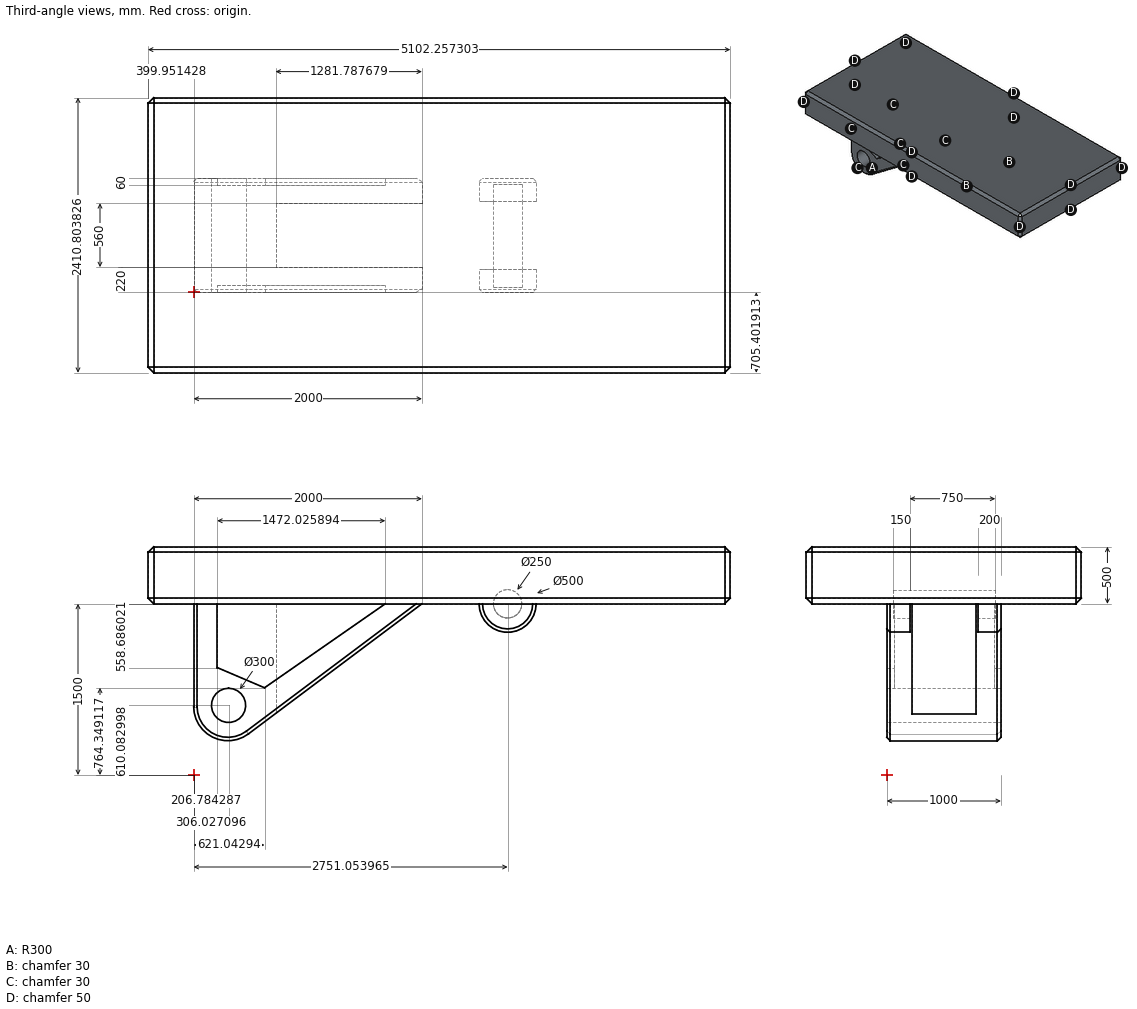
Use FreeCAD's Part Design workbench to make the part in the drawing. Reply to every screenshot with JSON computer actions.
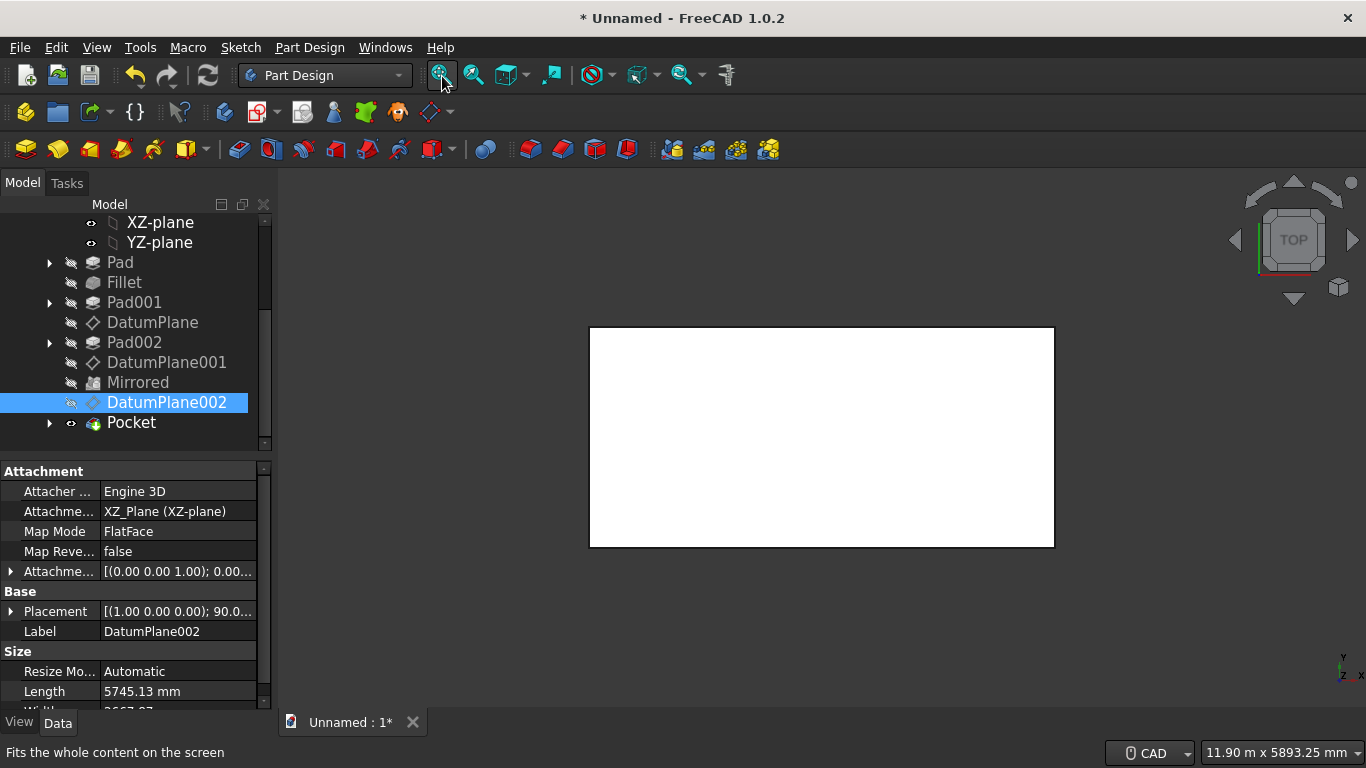
{"action": "key", "text": "0"}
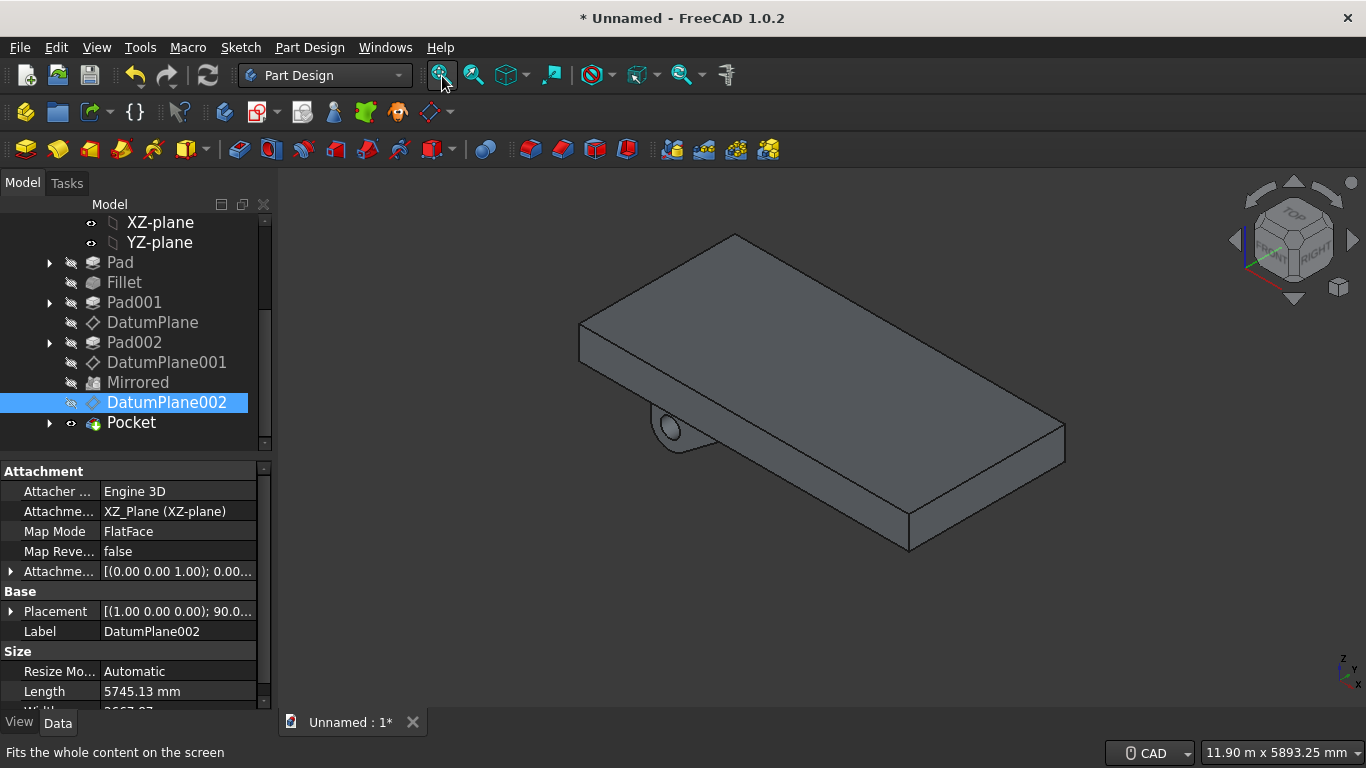
{"action": "key", "text": "1"}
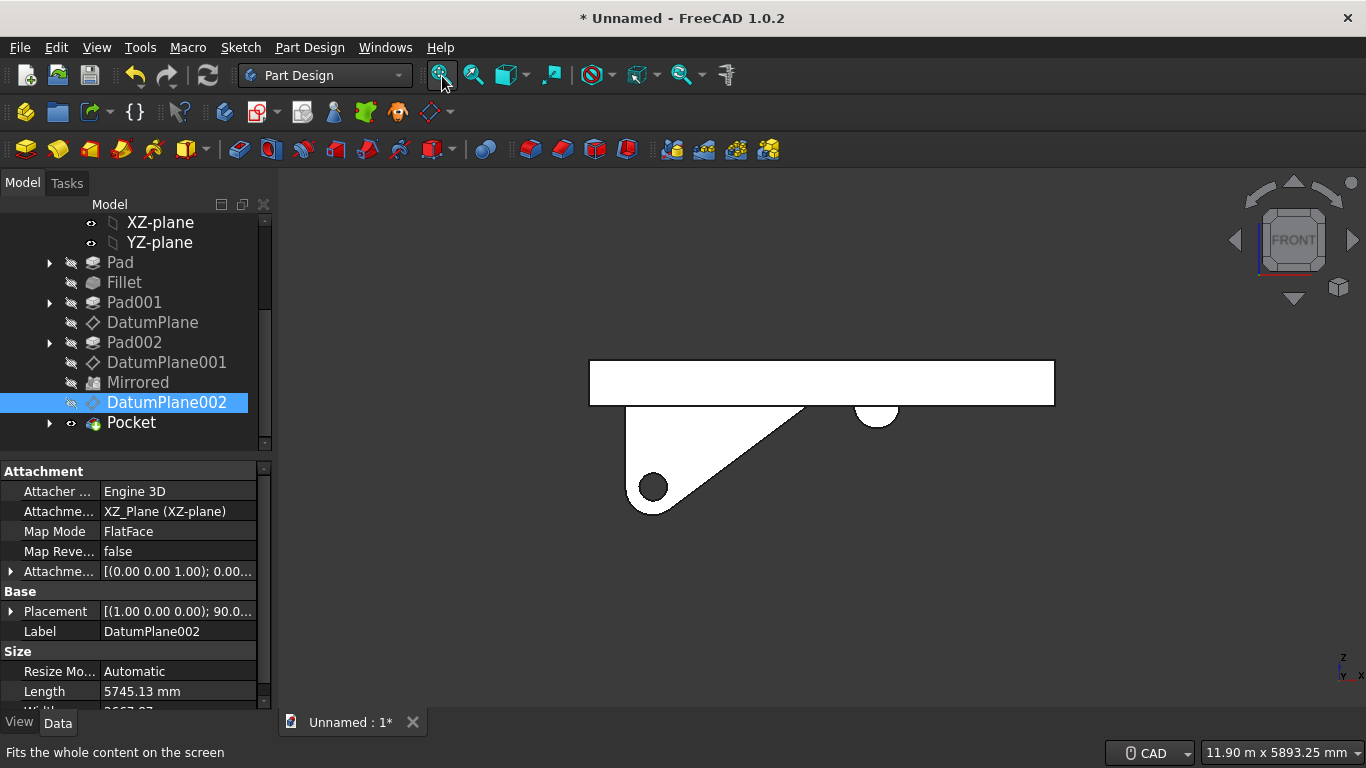
{"action": "left_click", "coordinate": [442, 76]}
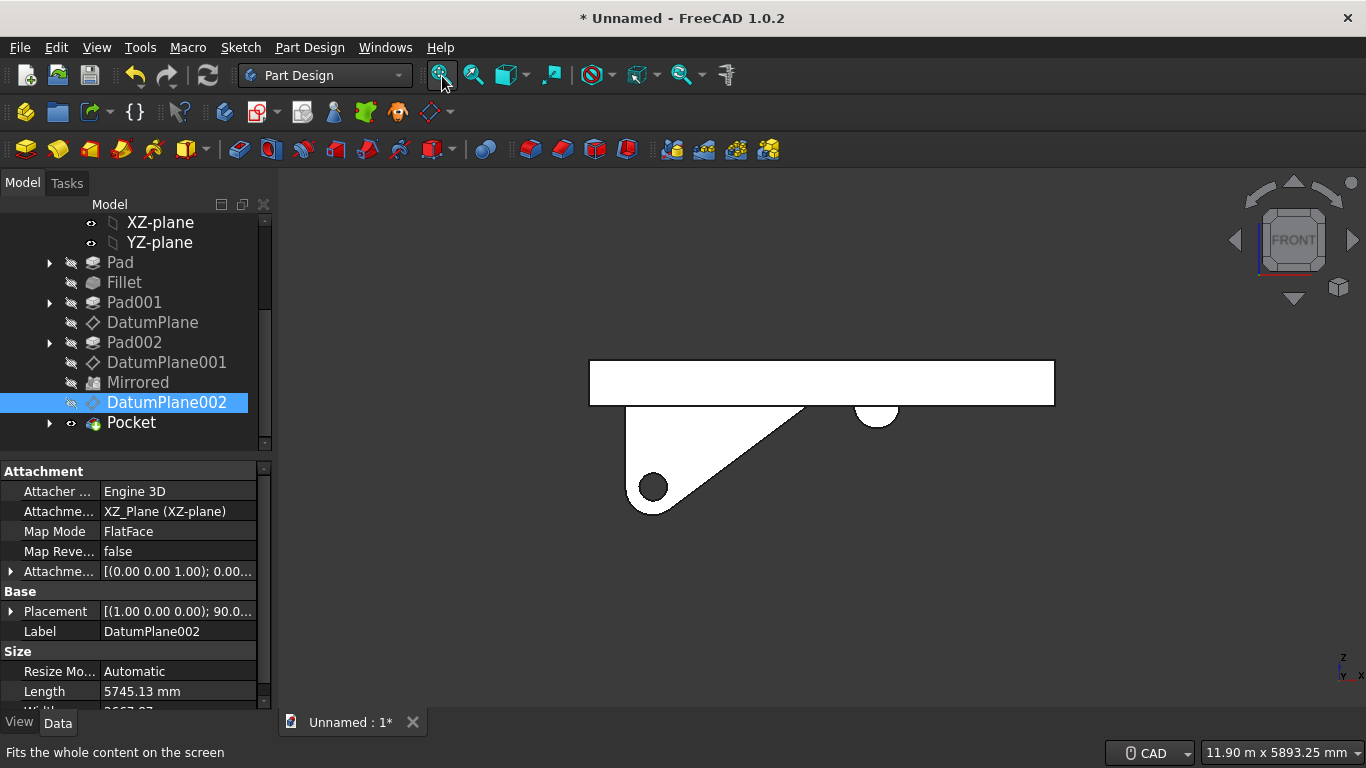
{"action": "left_click", "coordinate": [863, 423]}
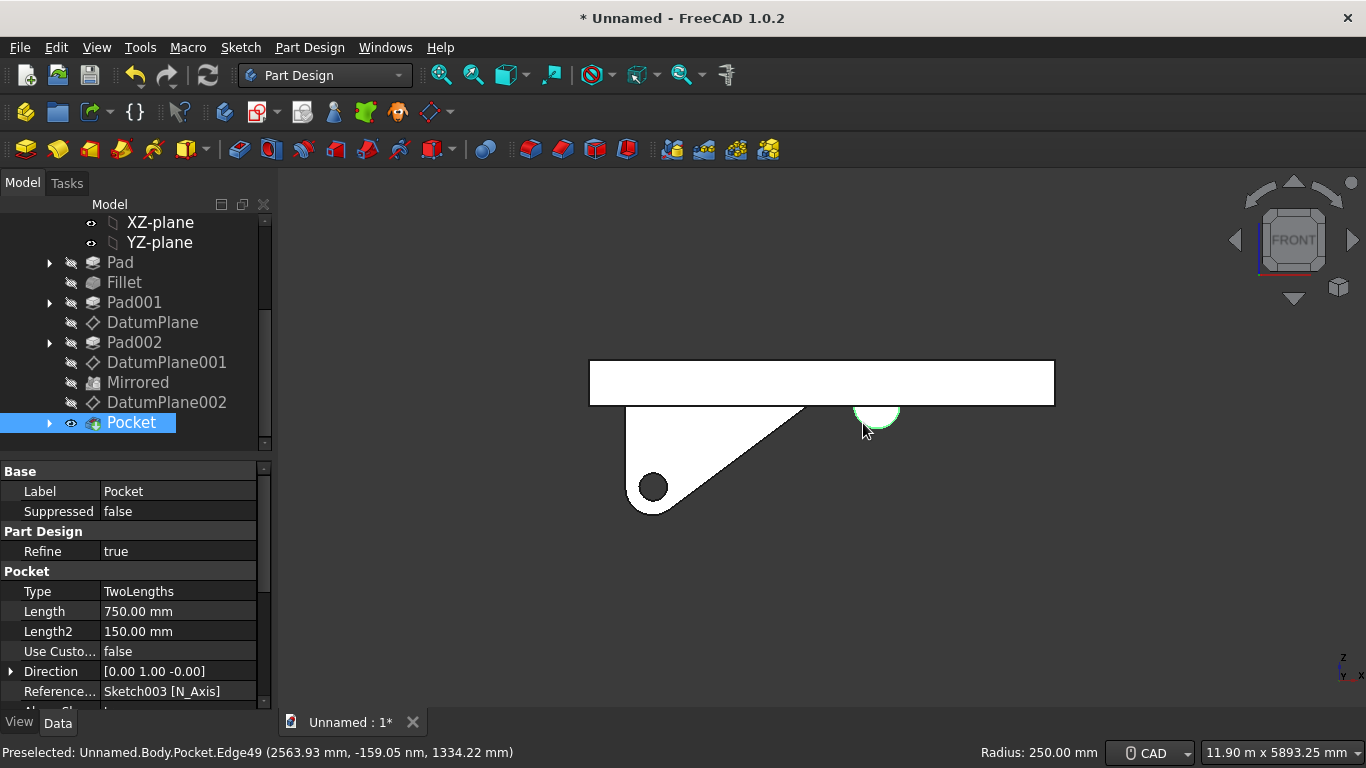
{"action": "key", "text": "3"}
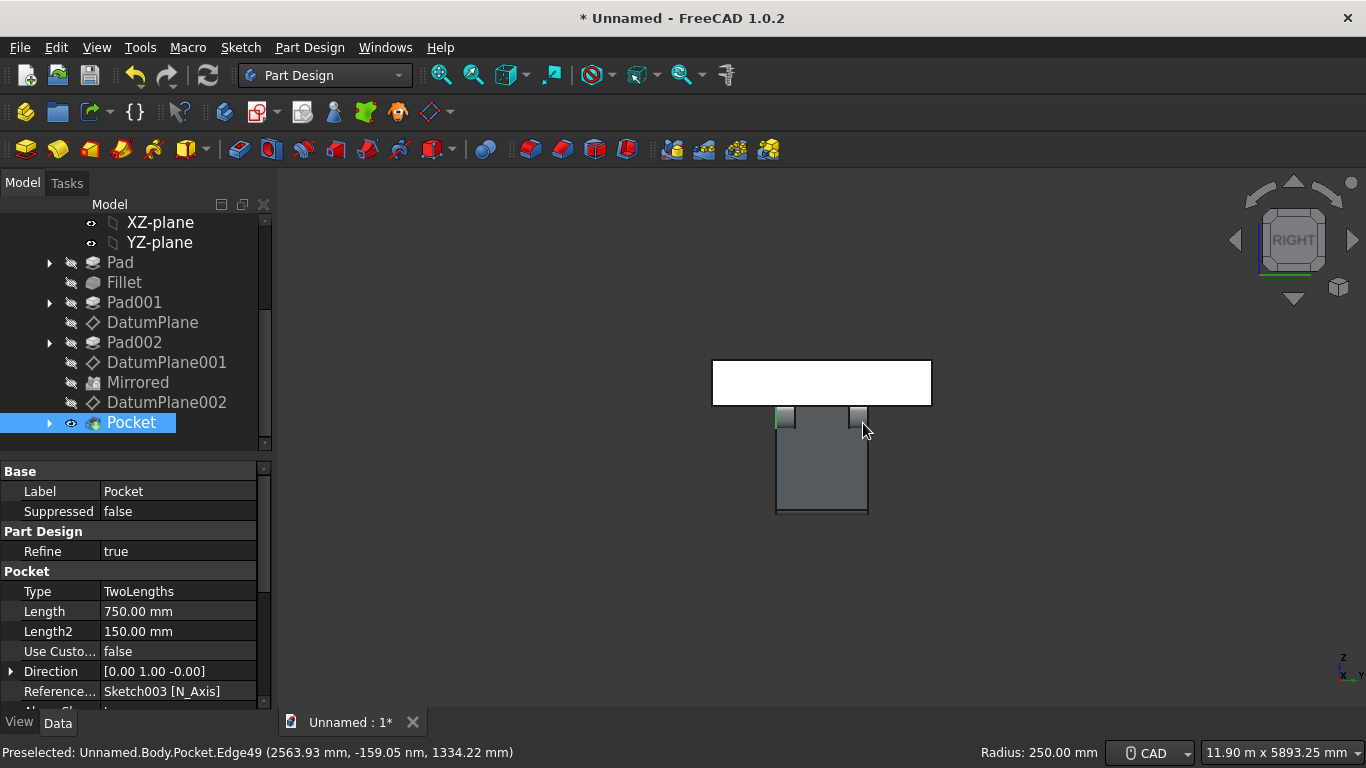
{"action": "key", "text": "v f"}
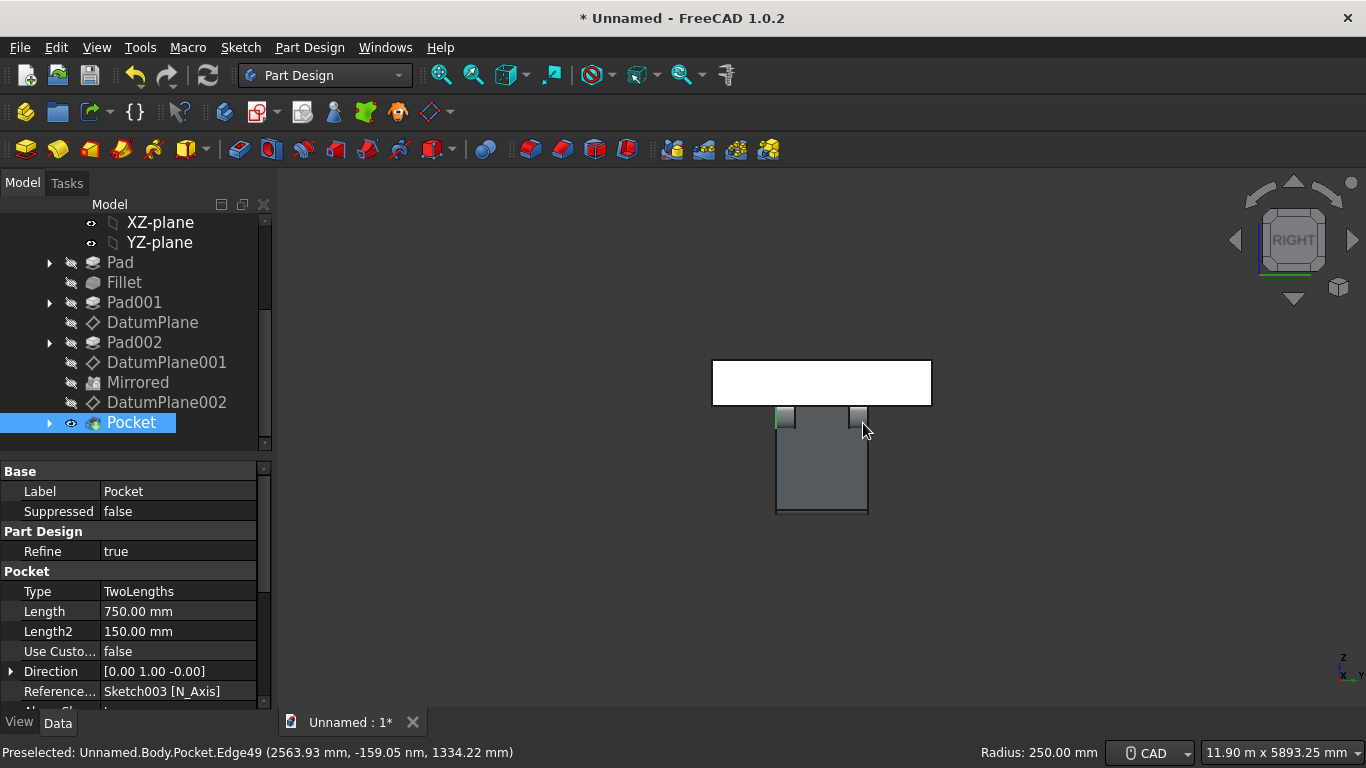
{"action": "left_click", "coordinate": [868, 427], "text": "ctrl"}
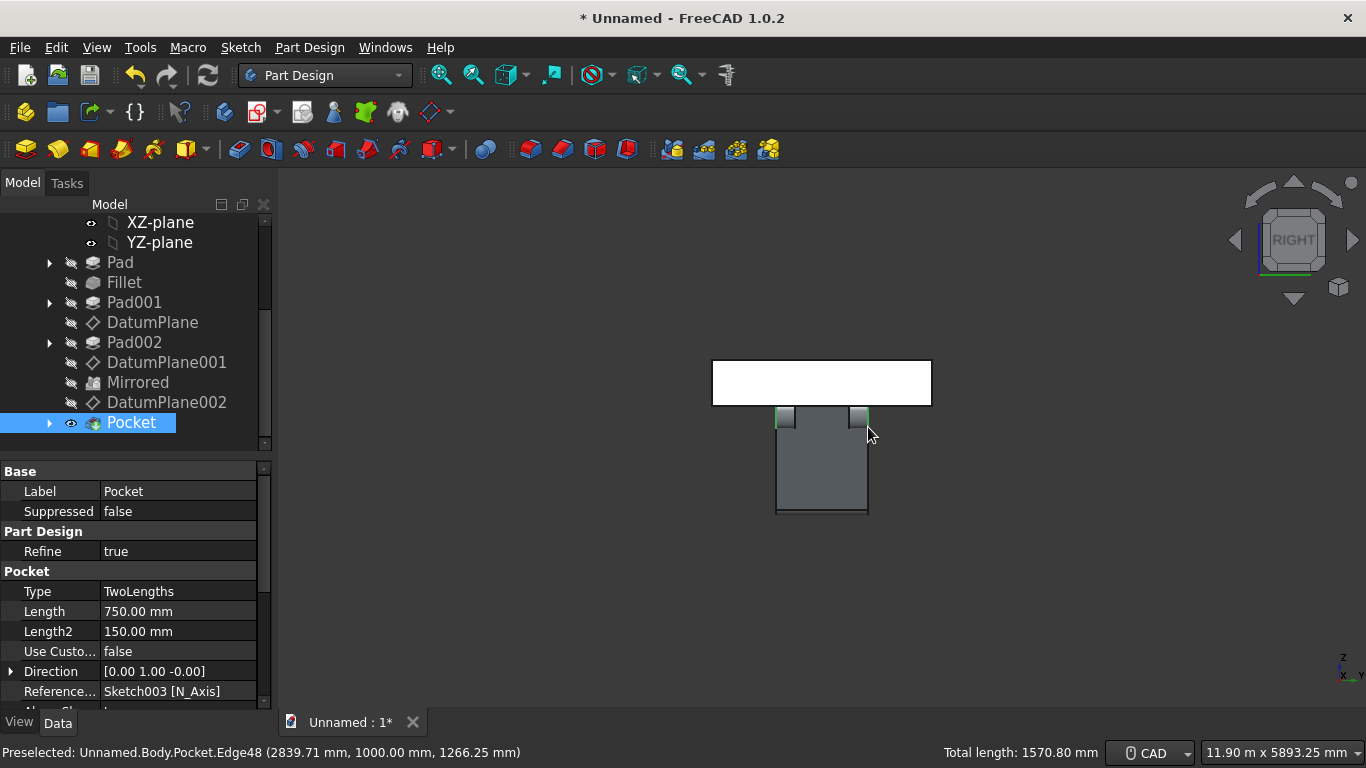
{"action": "left_click", "coordinate": [564, 150]}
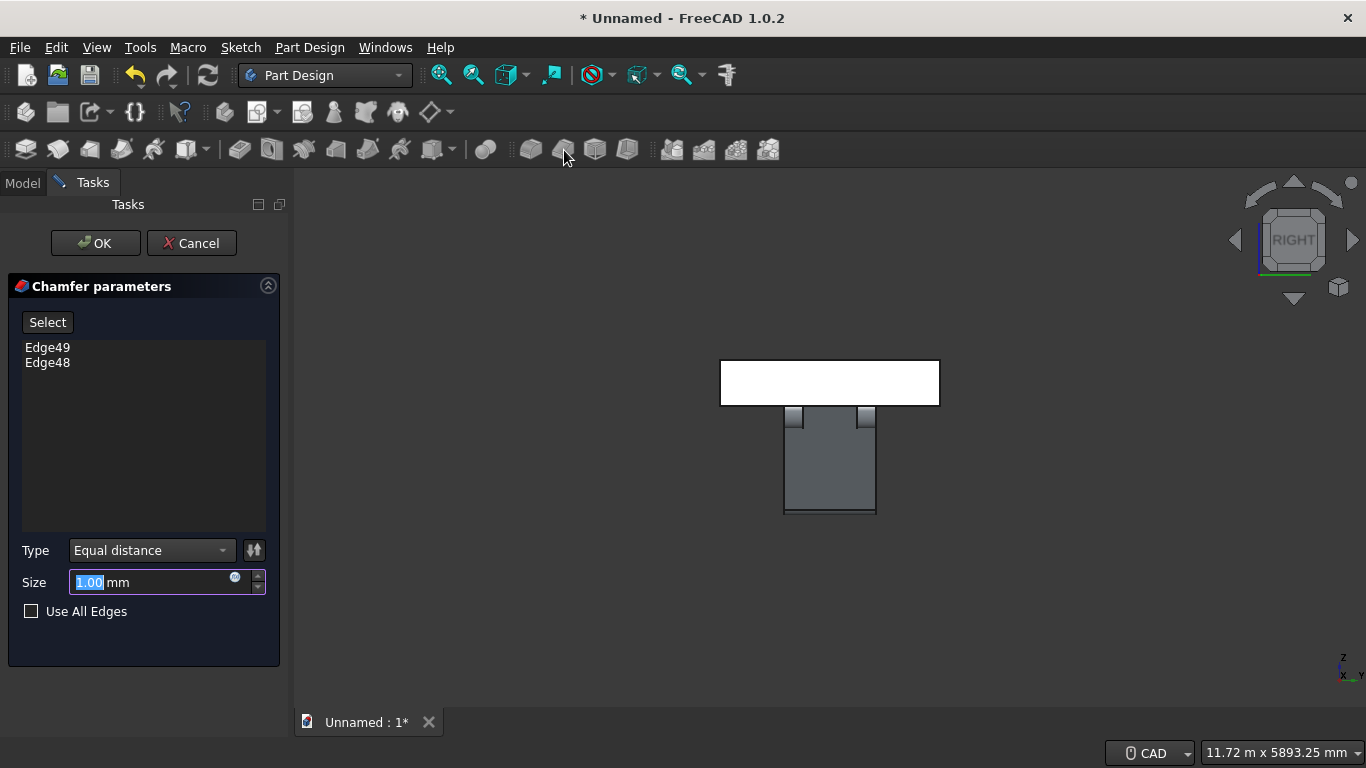
{"action": "type", "text": "30"}
{"action": "key", "text": "Tab"}